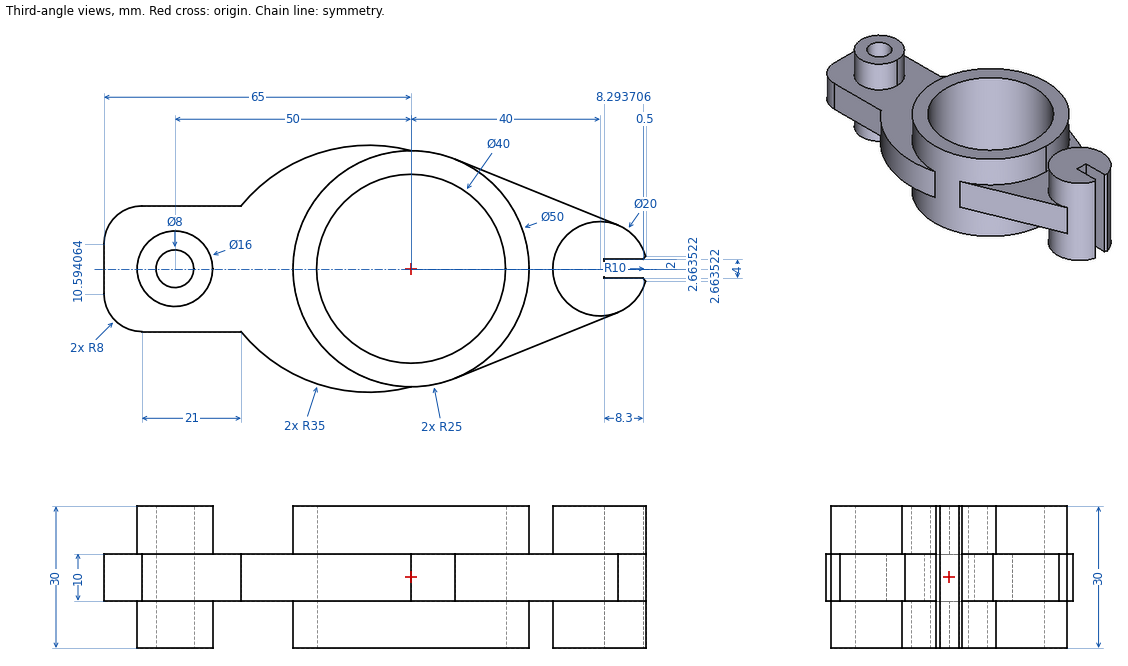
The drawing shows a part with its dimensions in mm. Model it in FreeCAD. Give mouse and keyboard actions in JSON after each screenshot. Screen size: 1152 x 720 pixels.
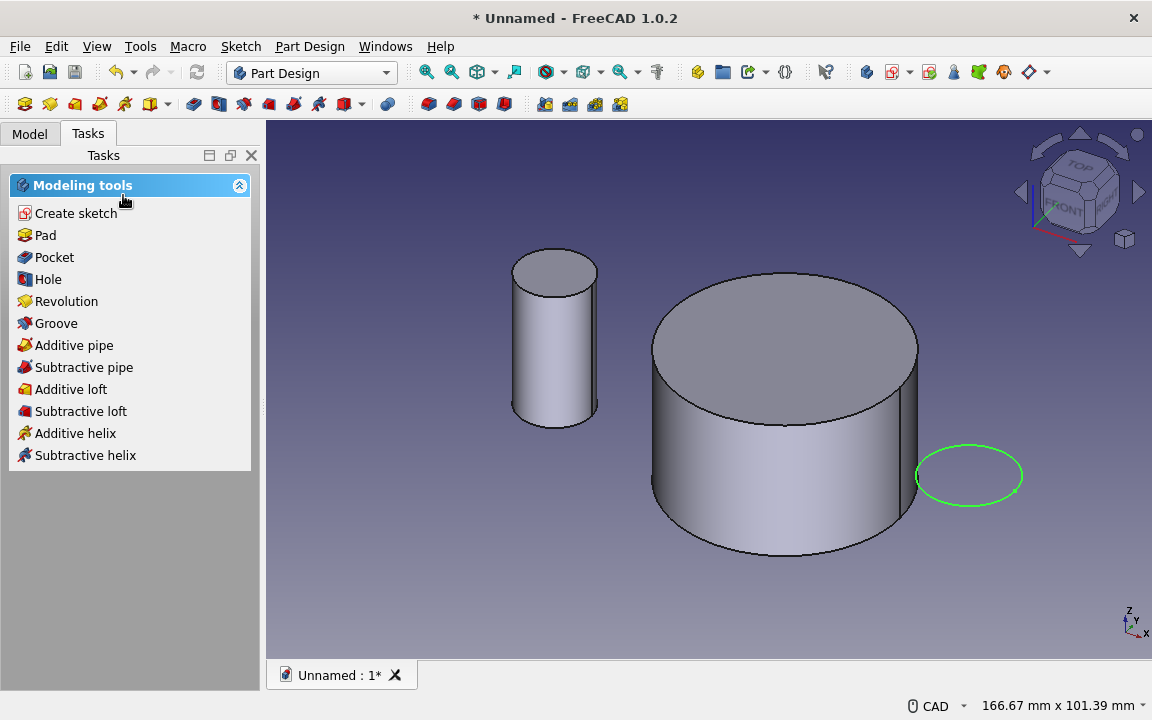
{"action": "left_click", "coordinate": [25, 104]}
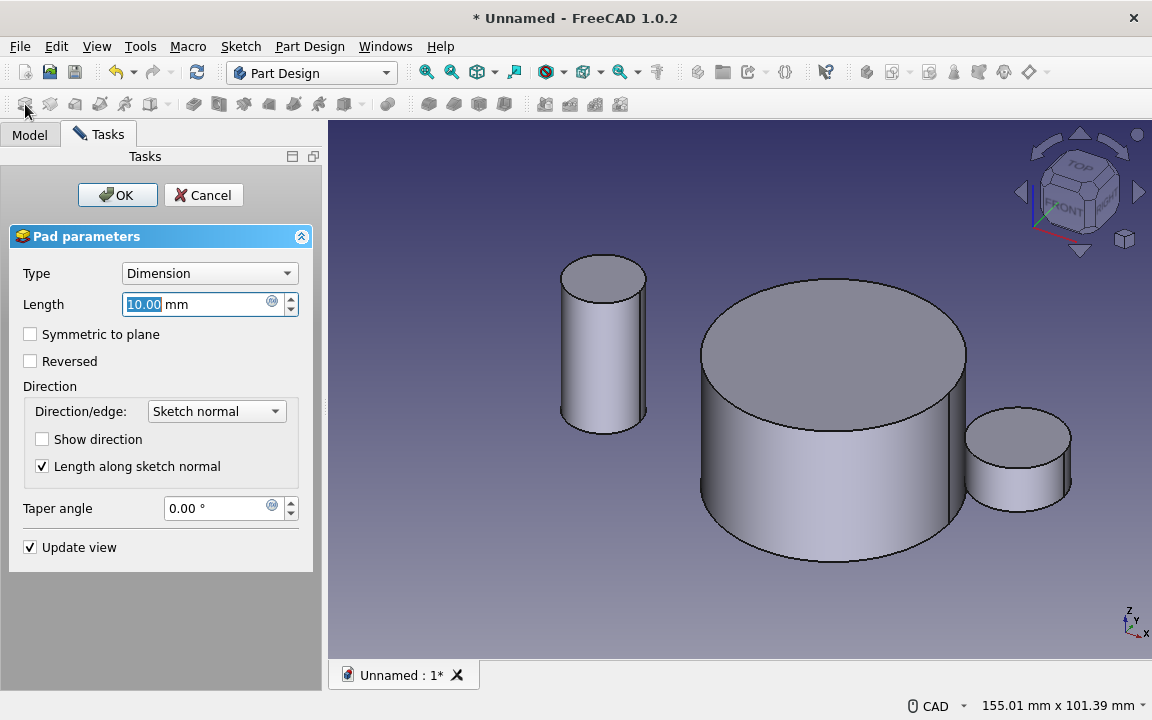
{"action": "type", "text": "30"}
{"action": "key", "text": "Tab"}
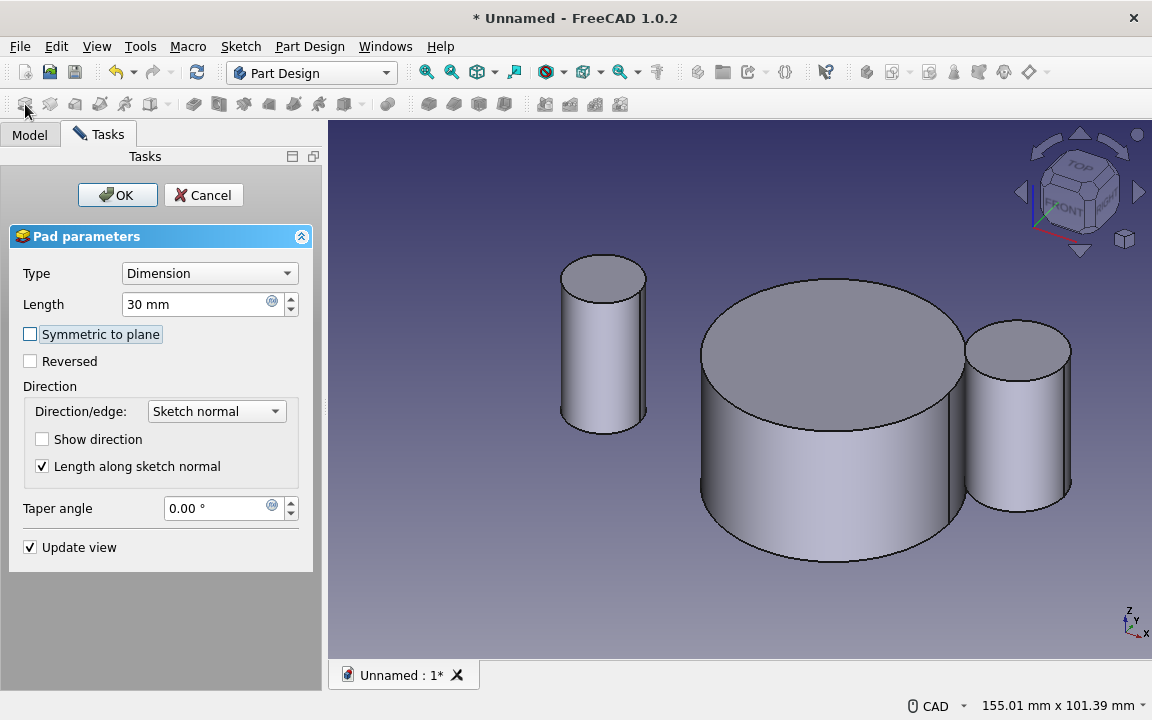
{"action": "left_click", "coordinate": [31, 334]}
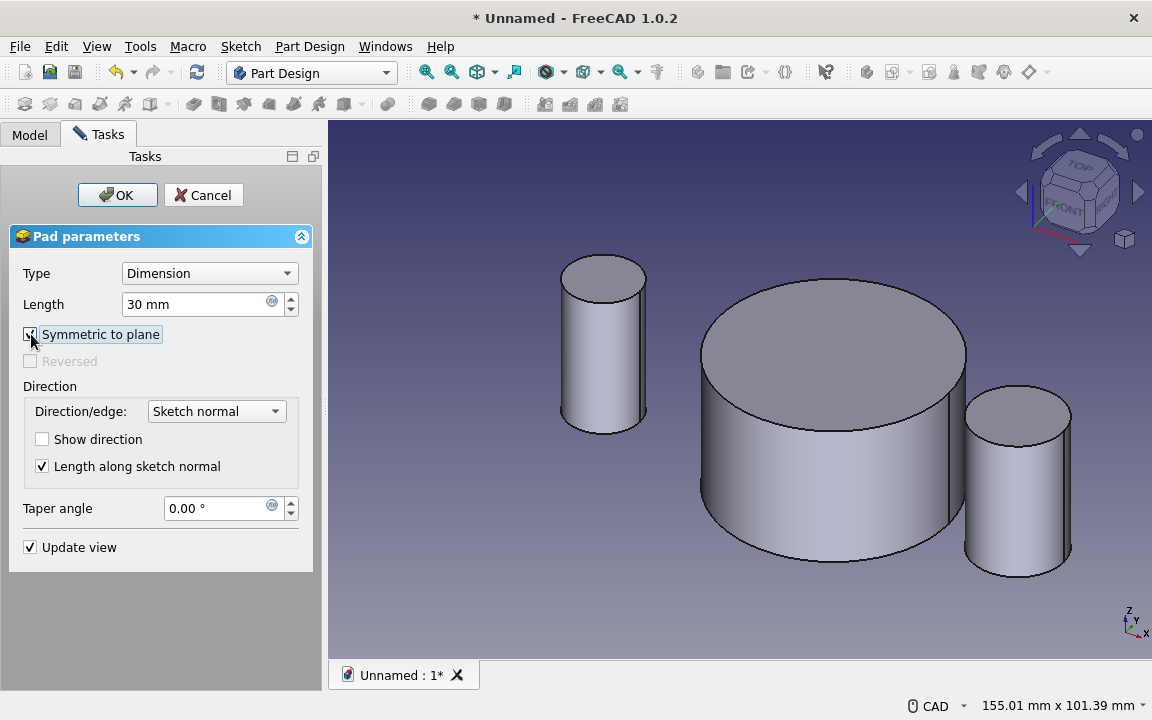
{"action": "left_click", "coordinate": [118, 195]}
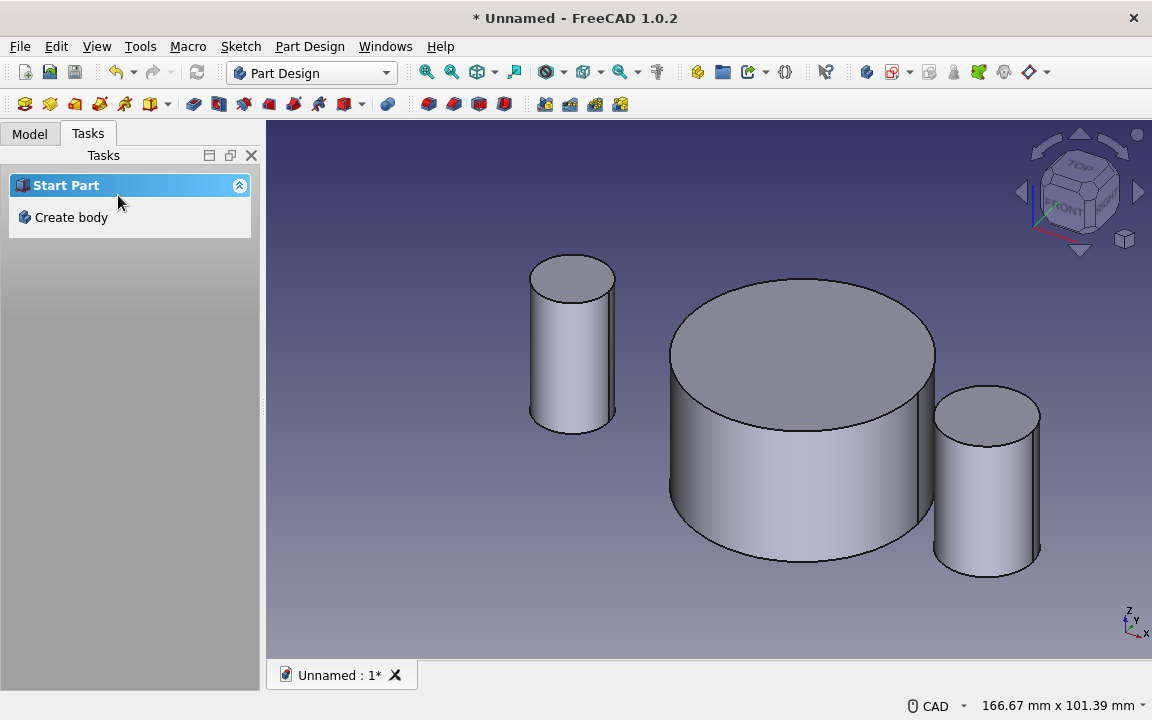
{"action": "left_click", "coordinate": [427, 72]}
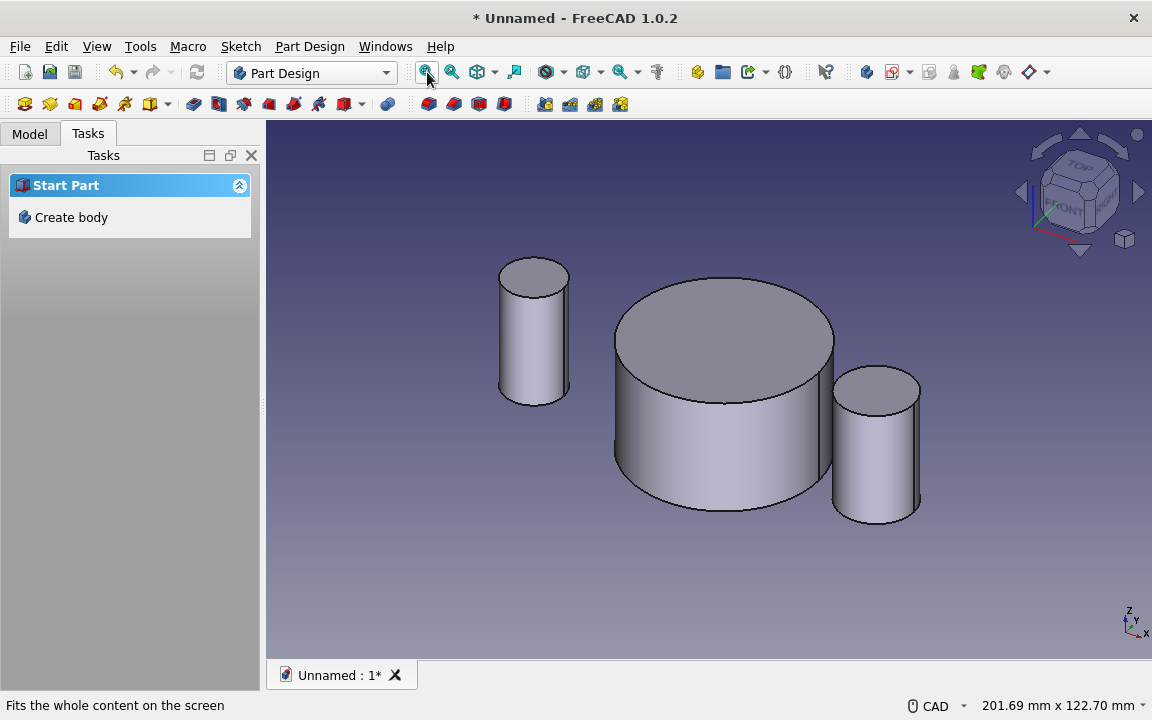
{"action": "left_click", "coordinate": [30, 134]}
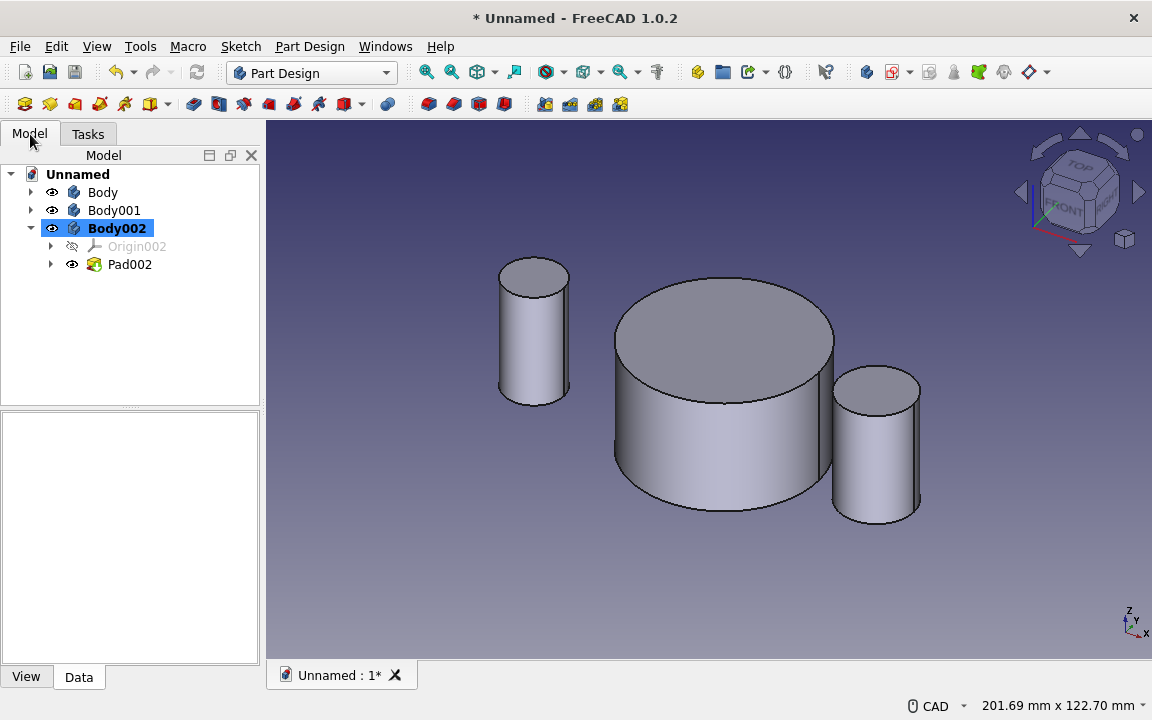
{"action": "double_click", "coordinate": [97, 192]}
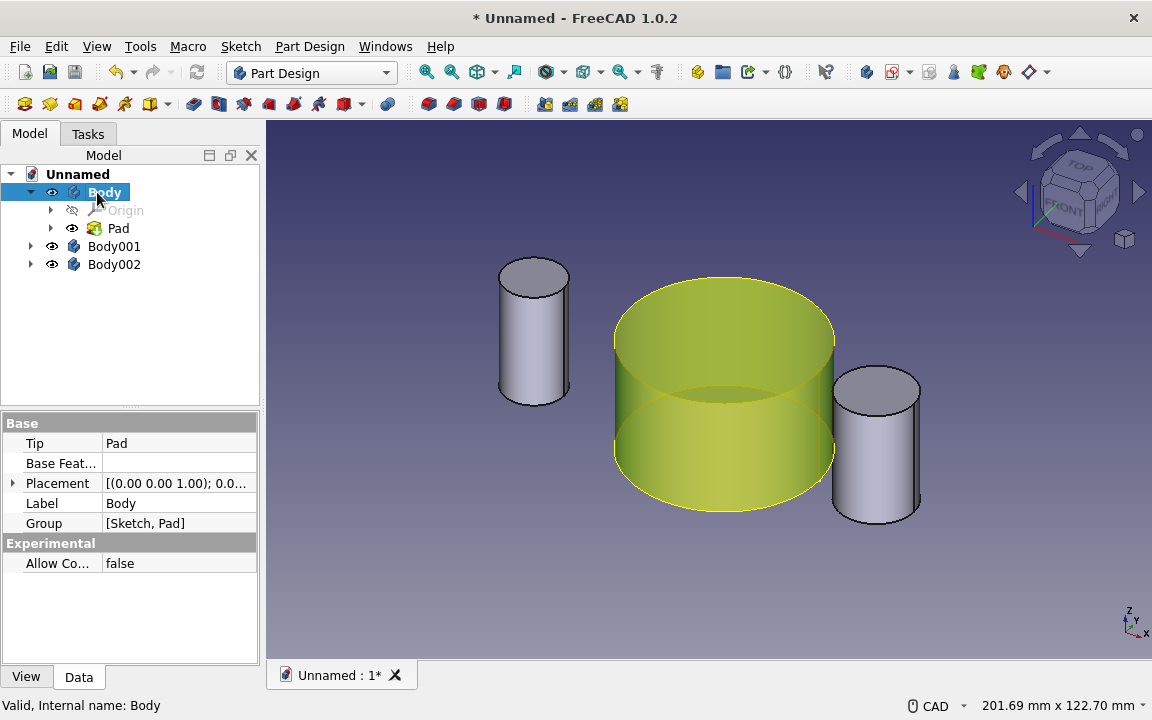
{"action": "left_click", "coordinate": [97, 192]}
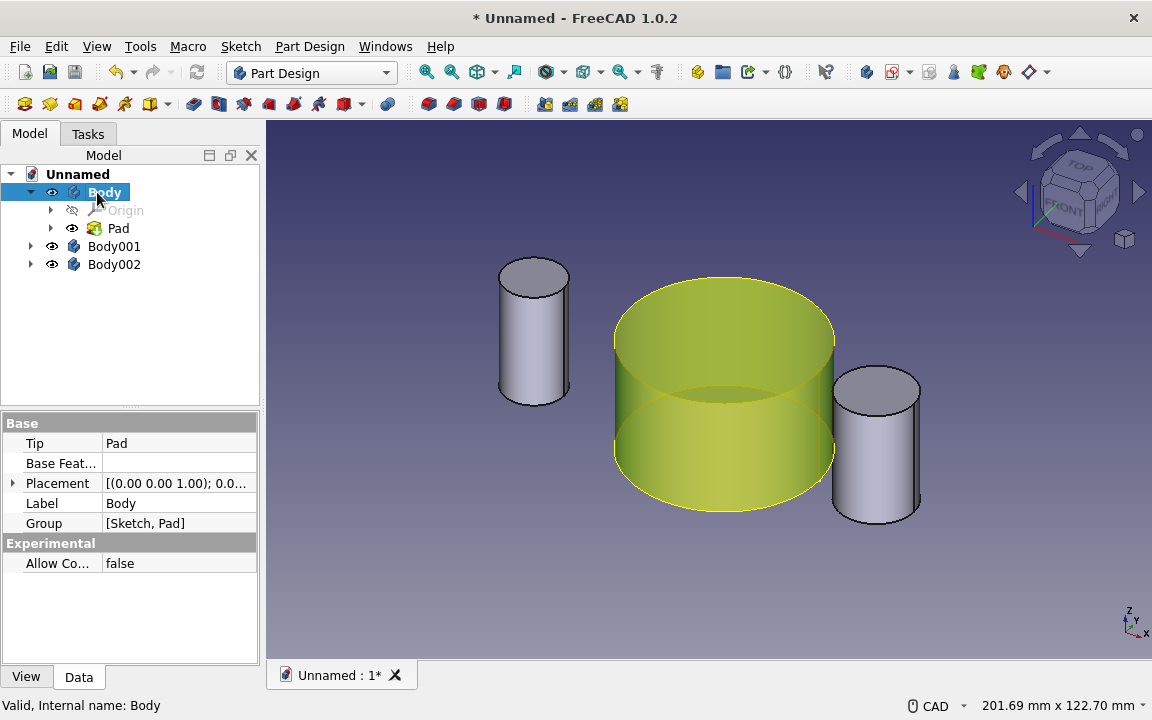
{"action": "left_click", "coordinate": [148, 563]}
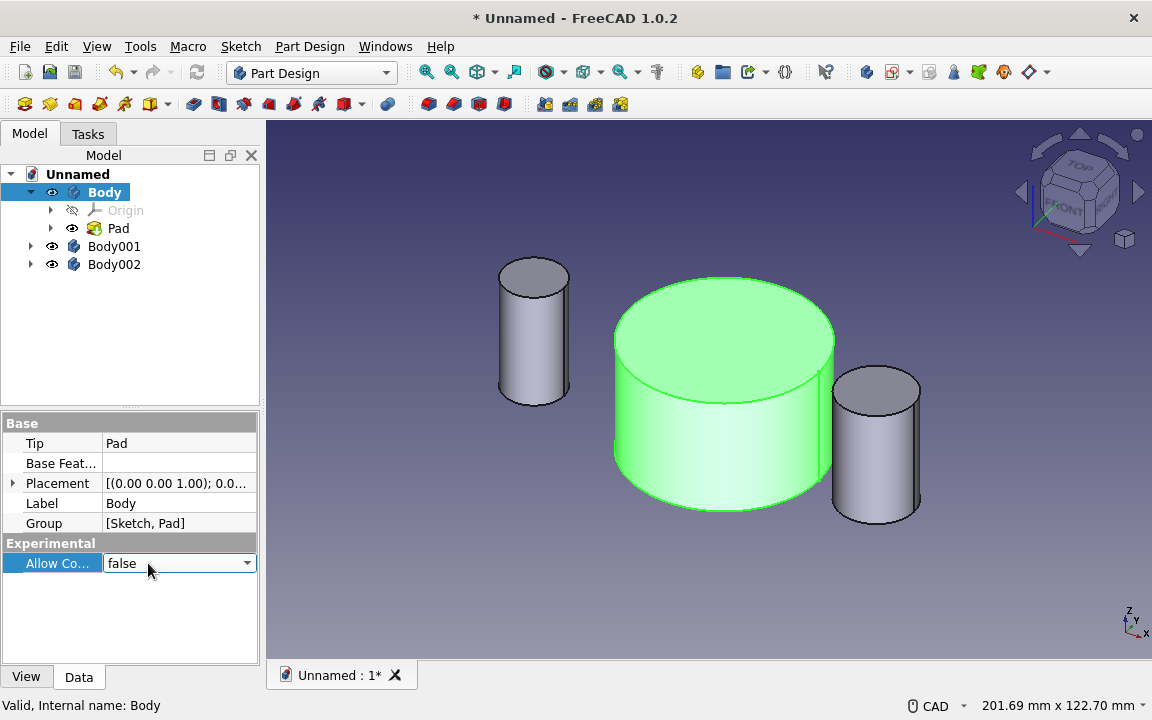
{"action": "left_click", "coordinate": [148, 563]}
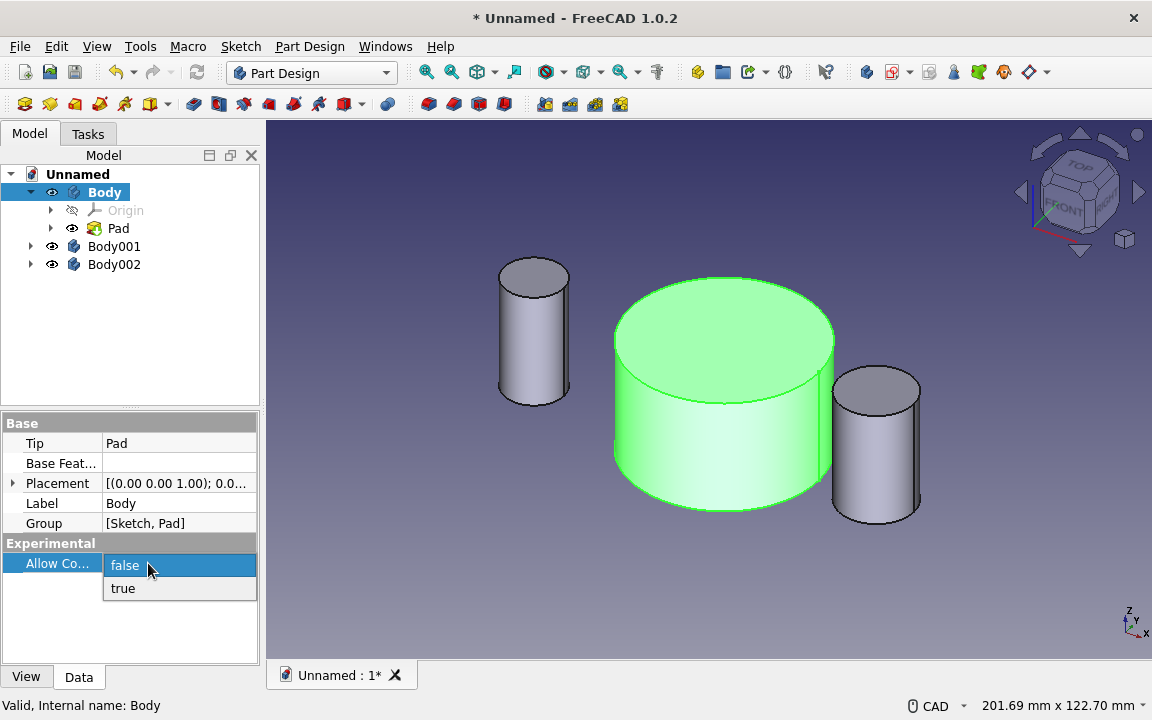
{"action": "left_click", "coordinate": [178, 588]}
{"action": "key", "text": "Return"}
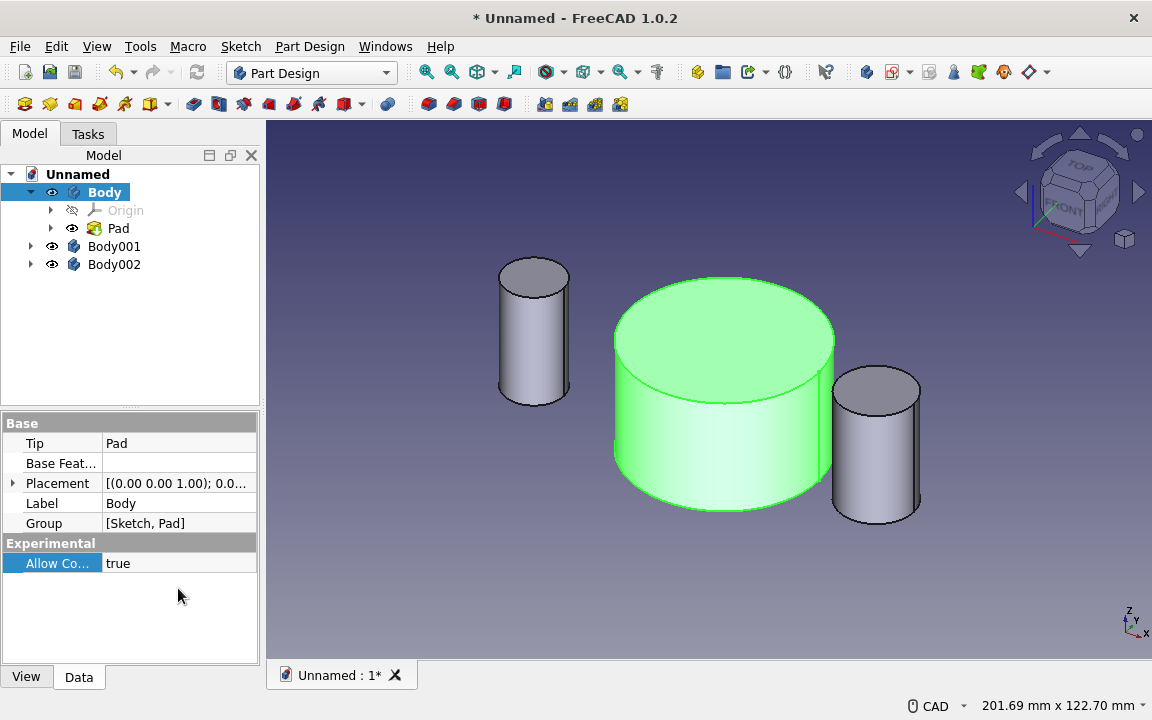
{"action": "left_click", "coordinate": [97, 246]}